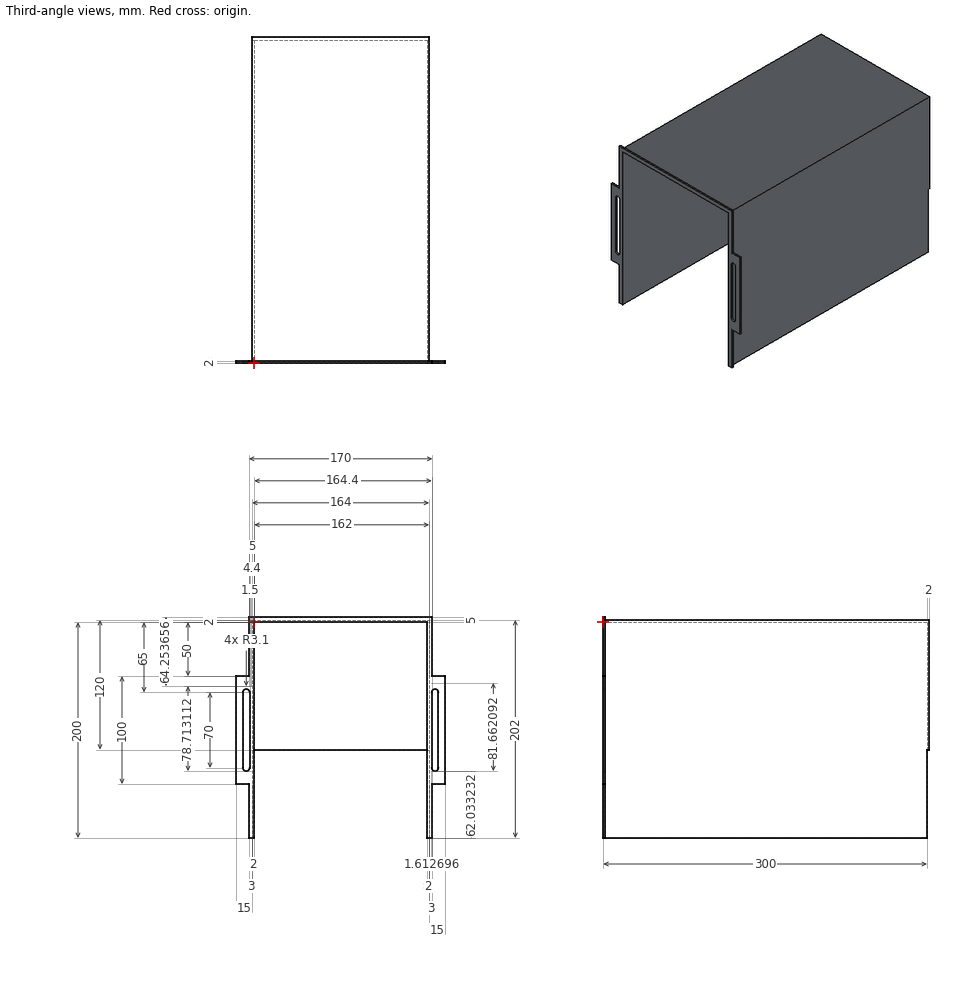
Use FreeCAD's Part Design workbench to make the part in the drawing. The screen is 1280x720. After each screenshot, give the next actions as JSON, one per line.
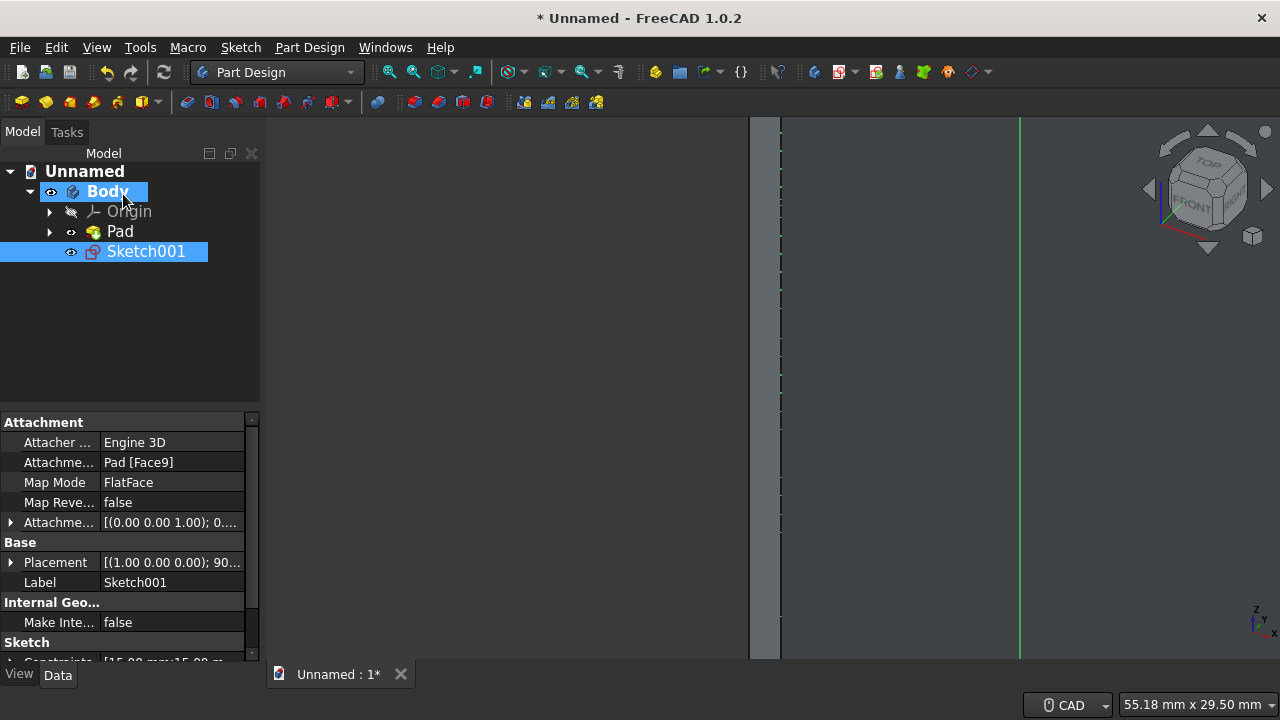
{"action": "left_click", "coordinate": [22, 102]}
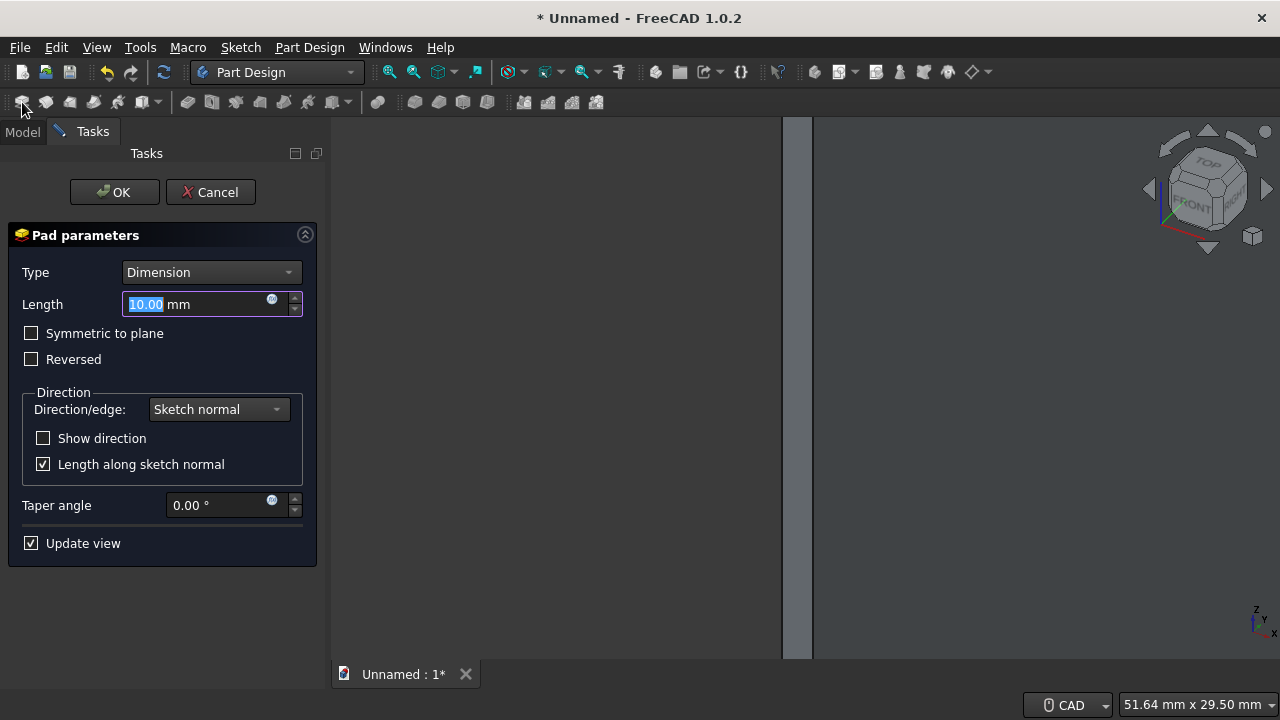
{"action": "type", "text": "2"}
{"action": "key", "text": "Tab"}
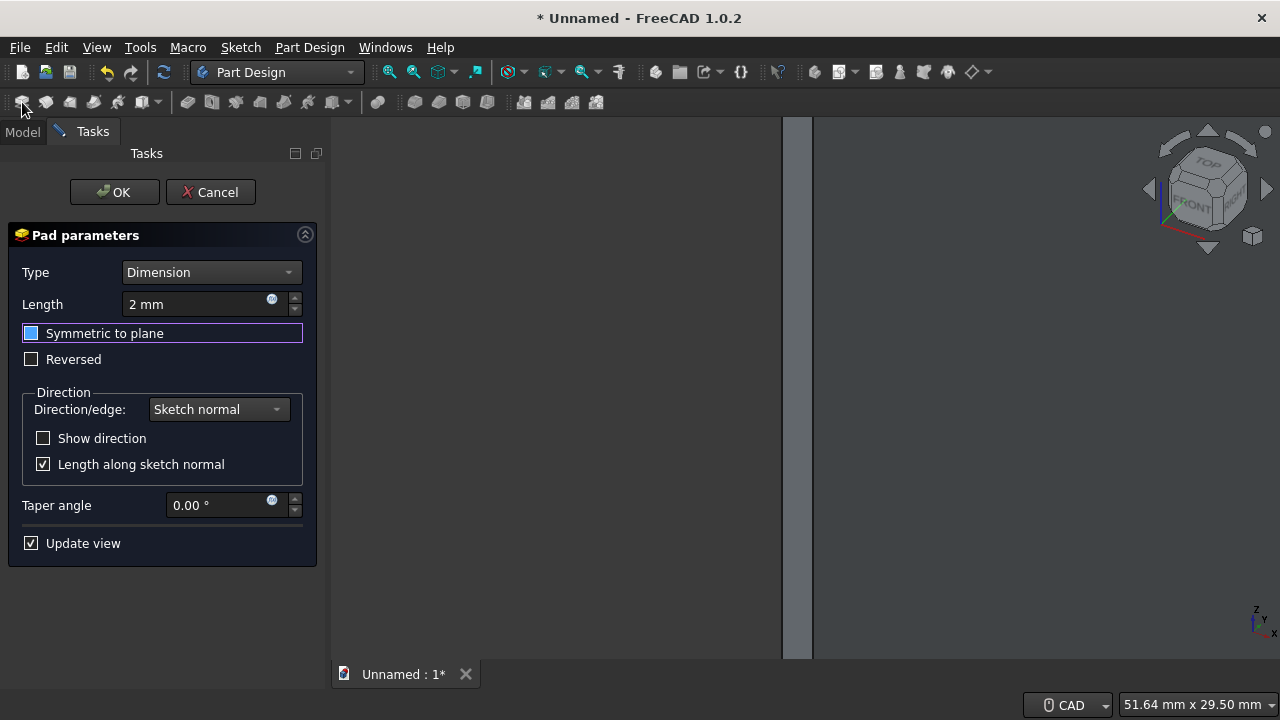
{"action": "left_click", "coordinate": [30, 359]}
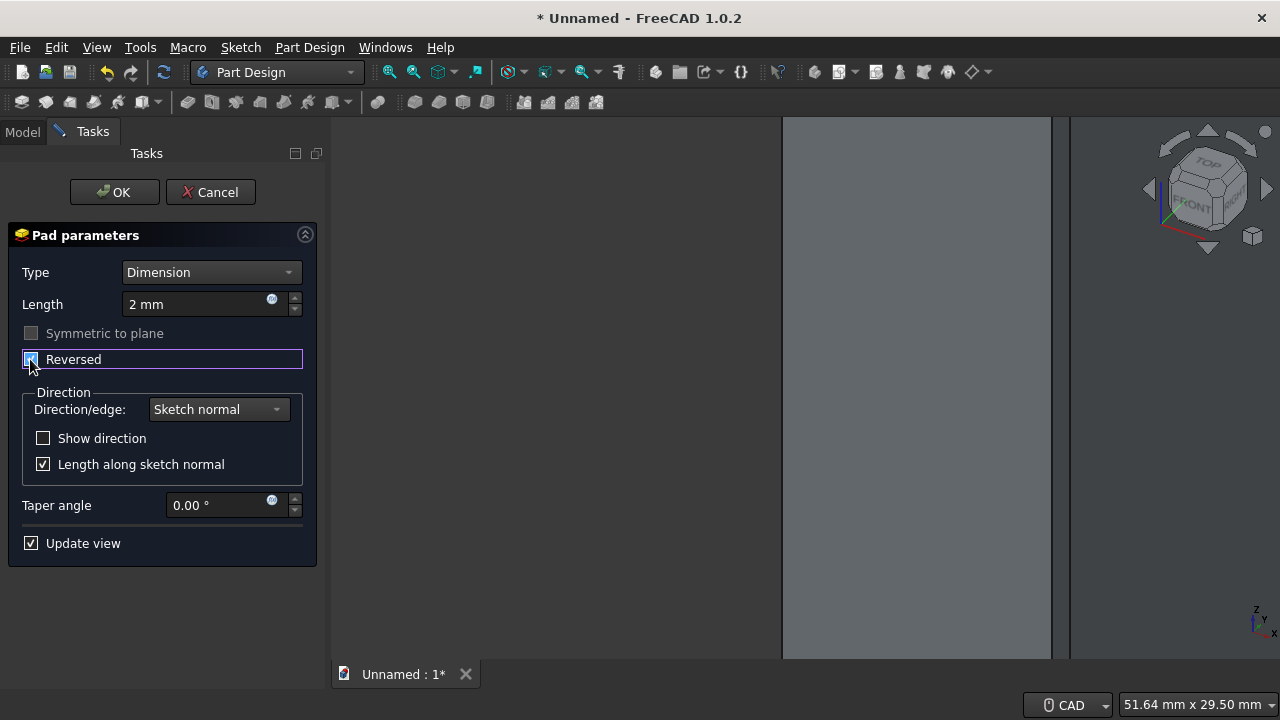
{"action": "left_click", "coordinate": [115, 192]}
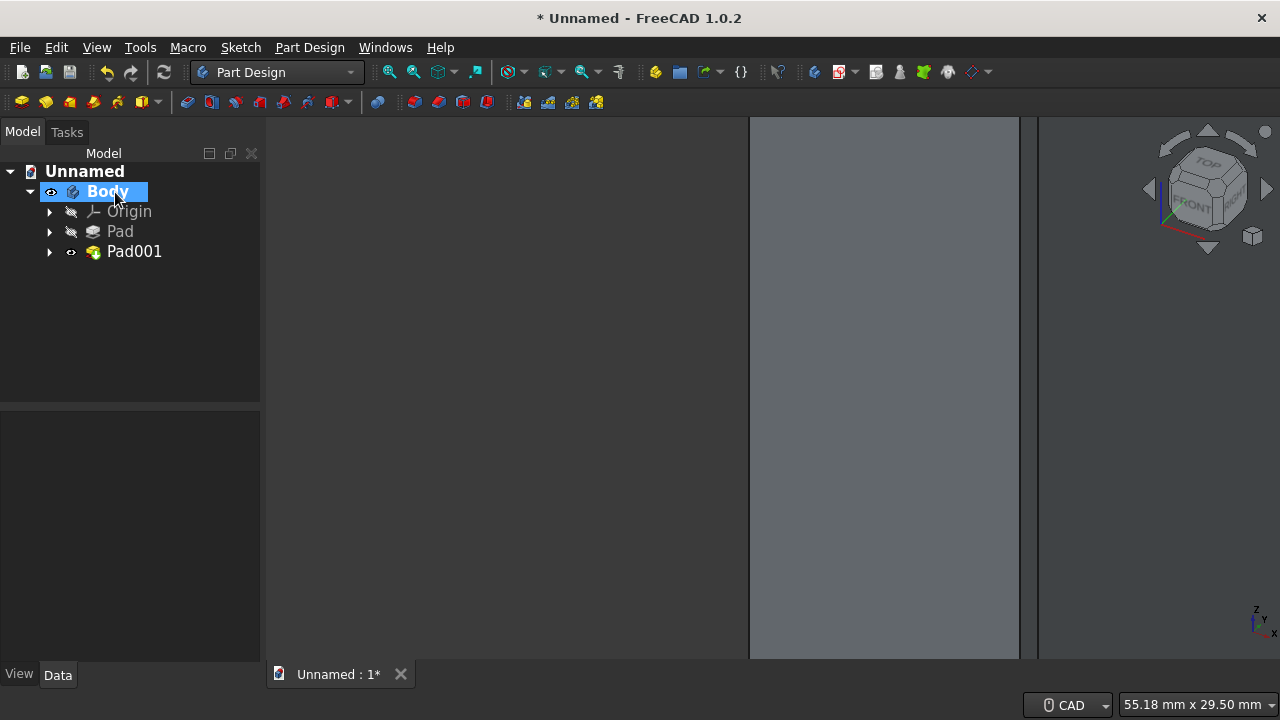
{"action": "left_click", "coordinate": [390, 72]}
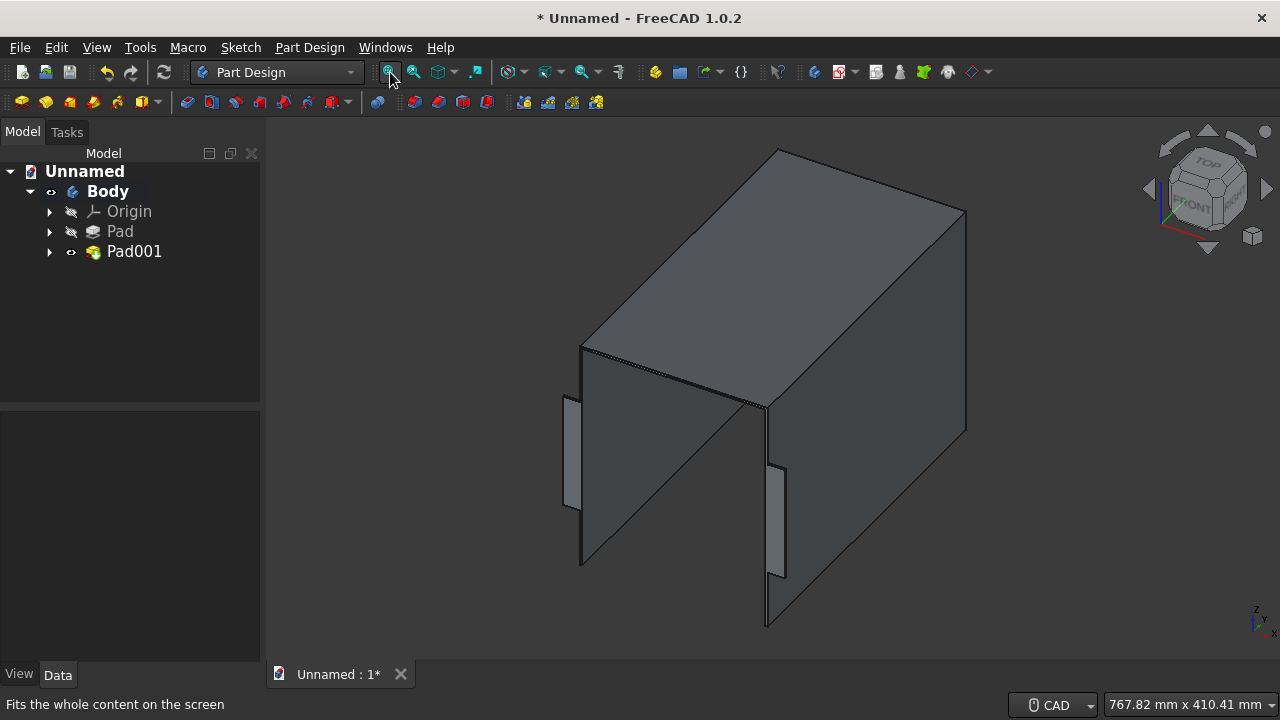
{"action": "left_click", "coordinate": [840, 72]}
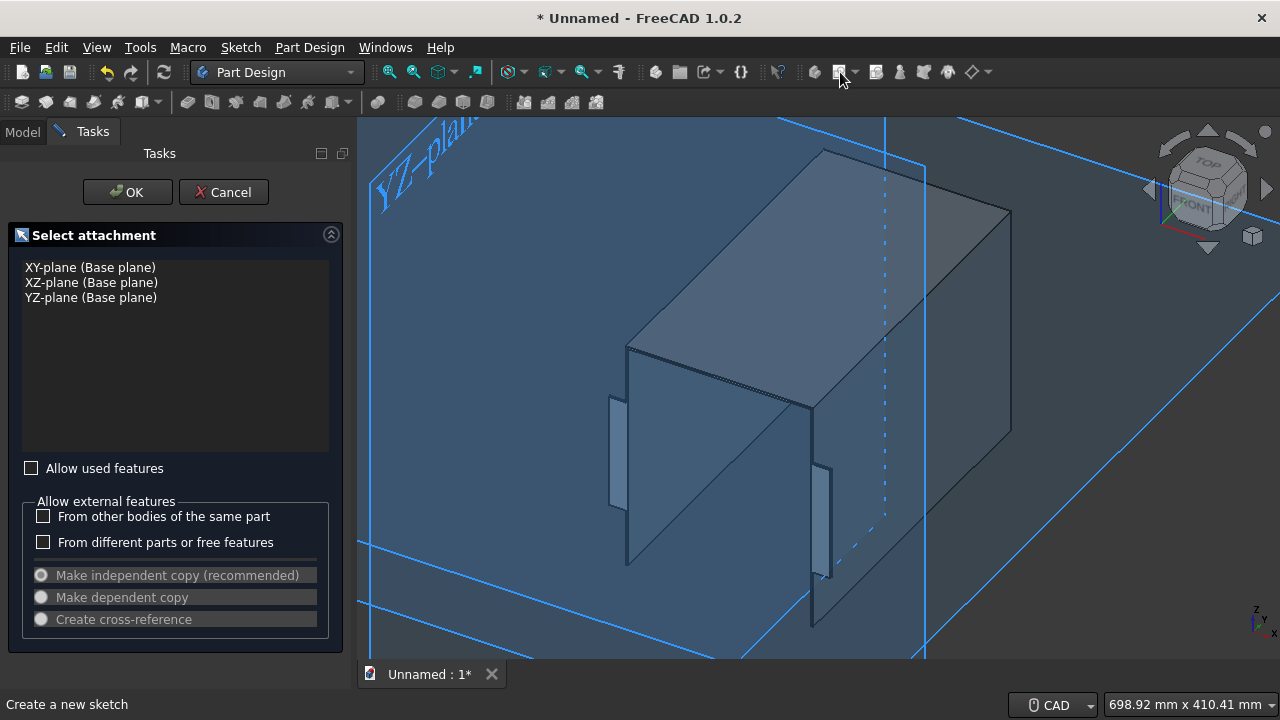
{"action": "left_click", "coordinate": [82, 282]}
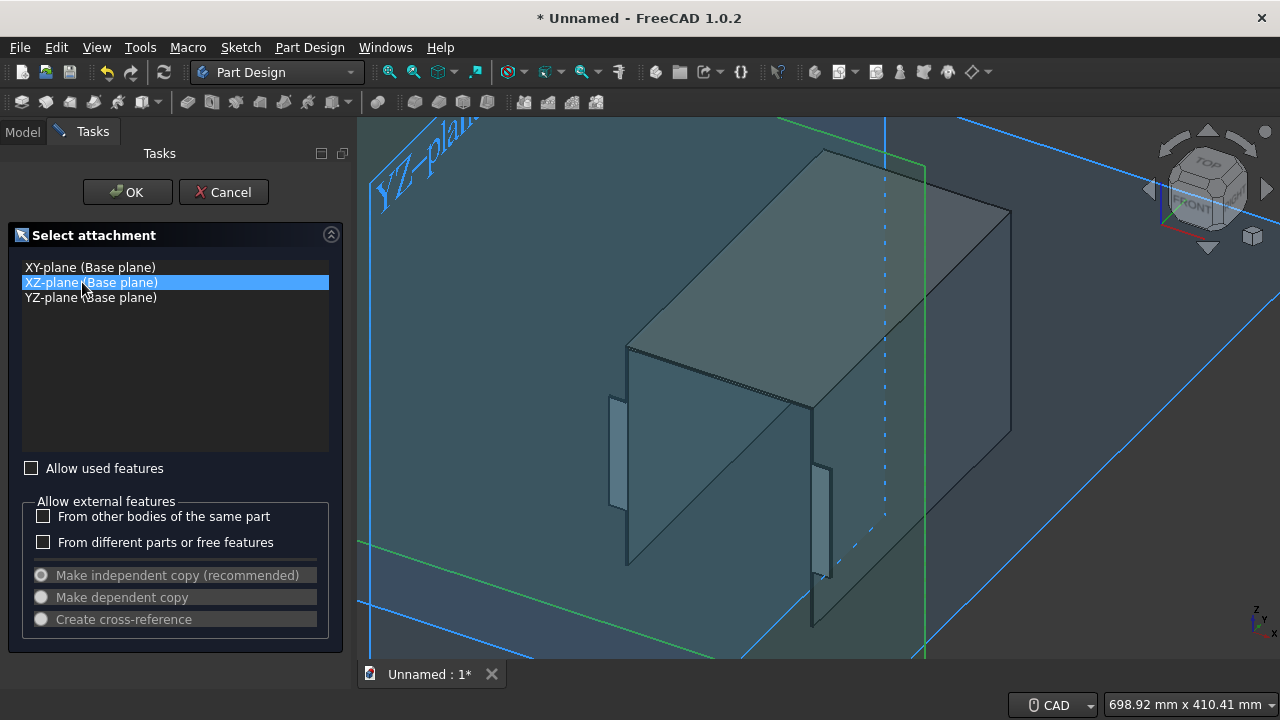
{"action": "left_click", "coordinate": [128, 192]}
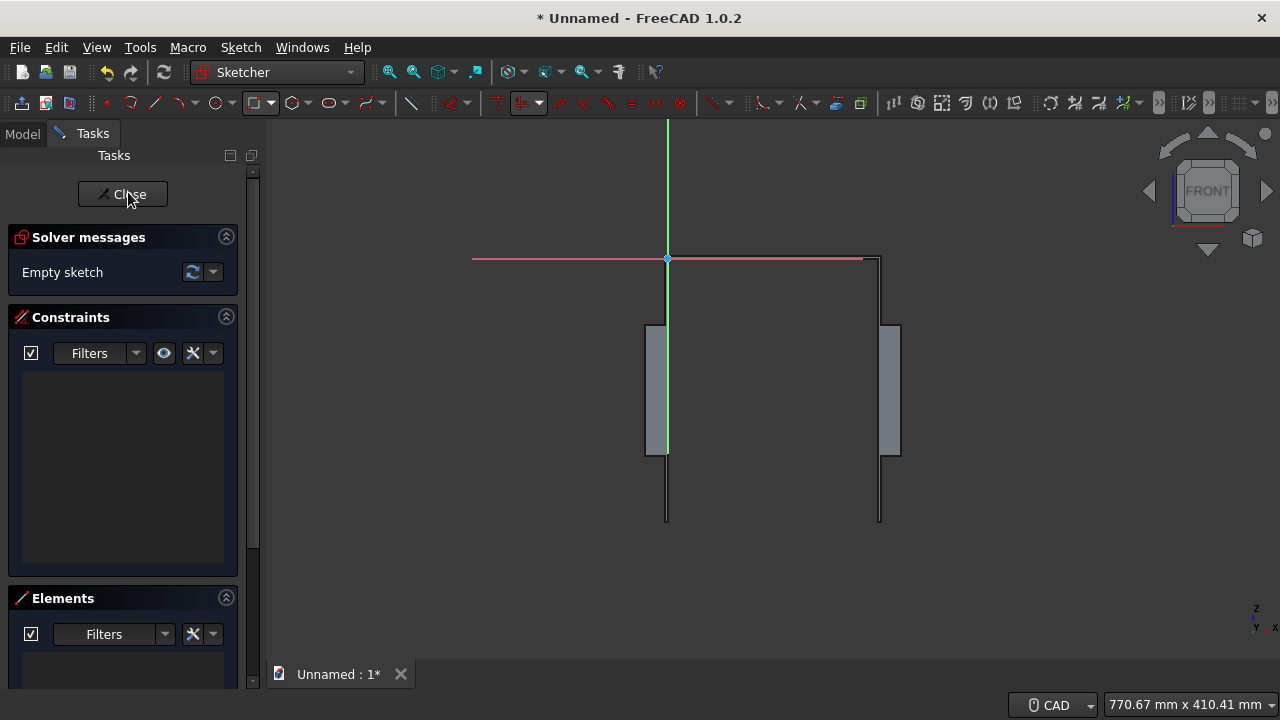
{"action": "scroll", "coordinate": [856, 302], "scroll_direction": "up", "scroll_amount": 3}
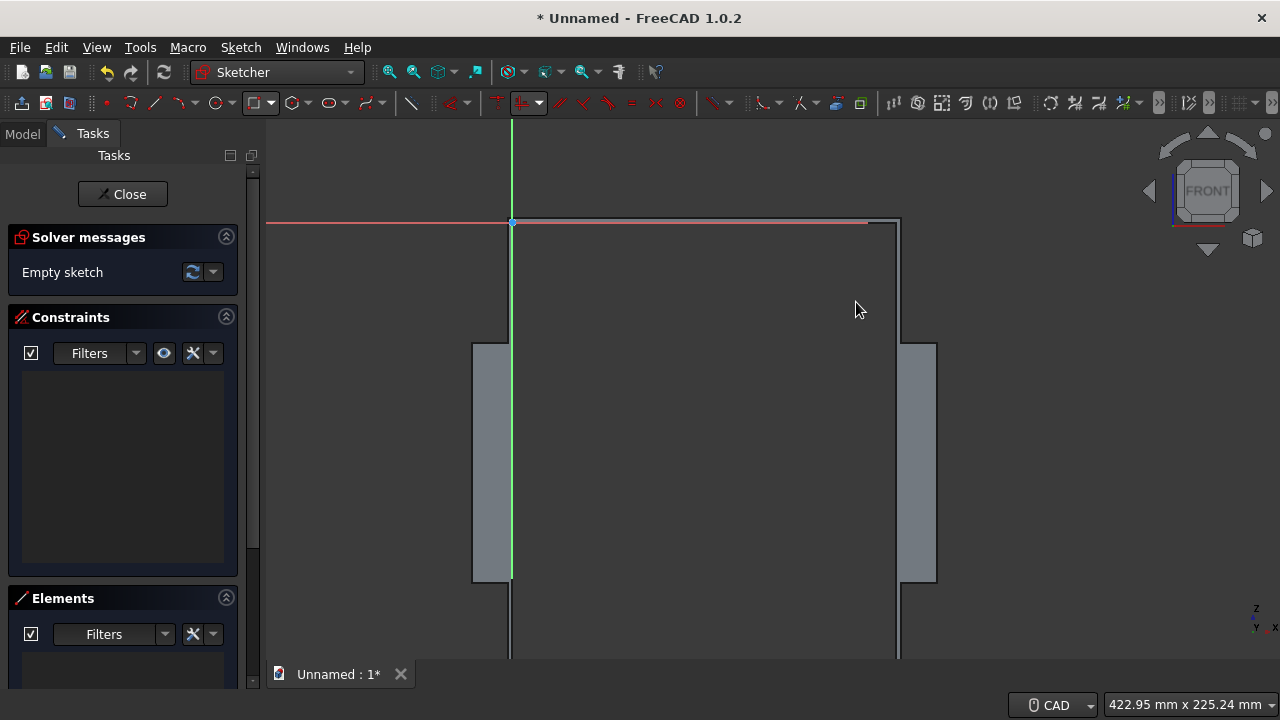
{"action": "left_click", "coordinate": [330, 104]}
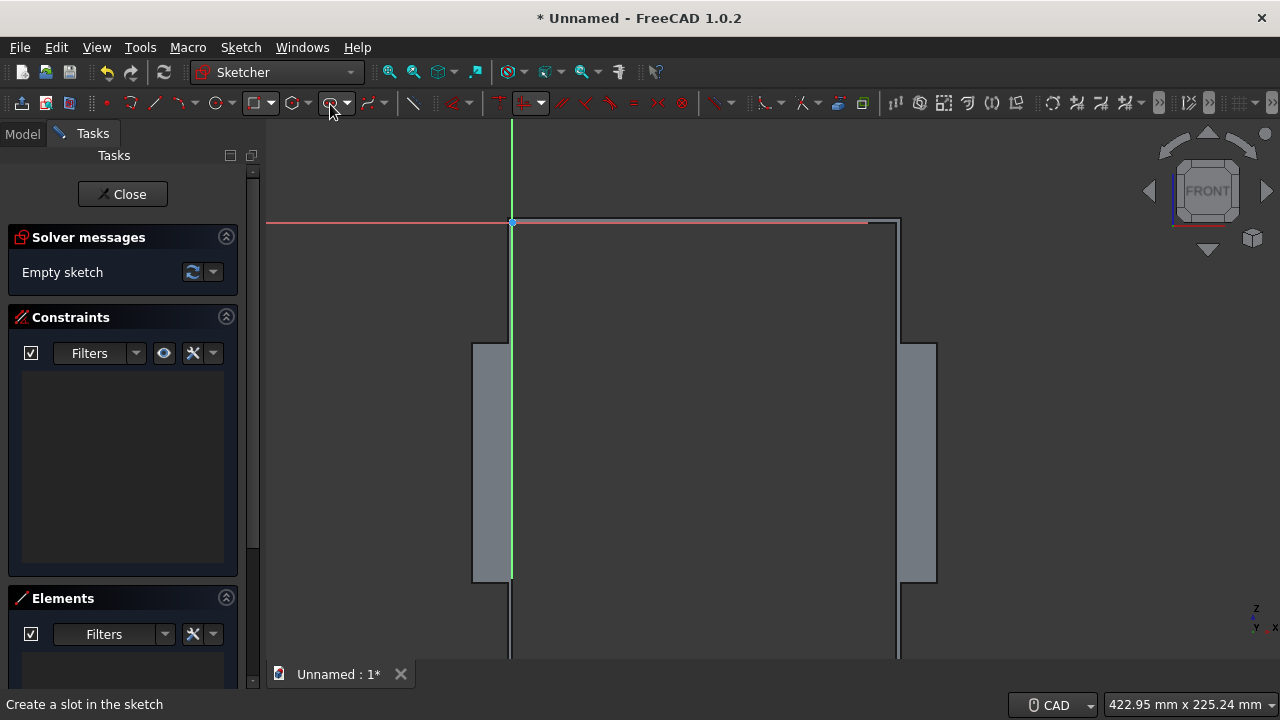
{"action": "scroll", "coordinate": [495, 547], "scroll_direction": "up", "scroll_amount": 6}